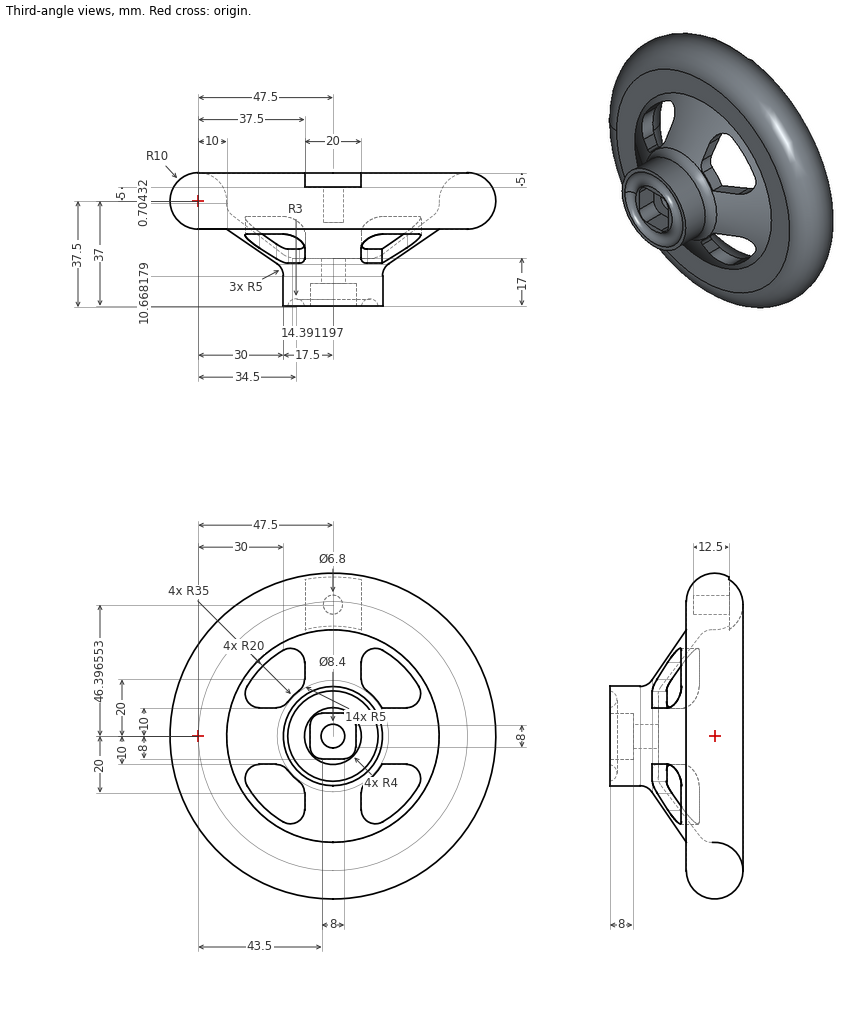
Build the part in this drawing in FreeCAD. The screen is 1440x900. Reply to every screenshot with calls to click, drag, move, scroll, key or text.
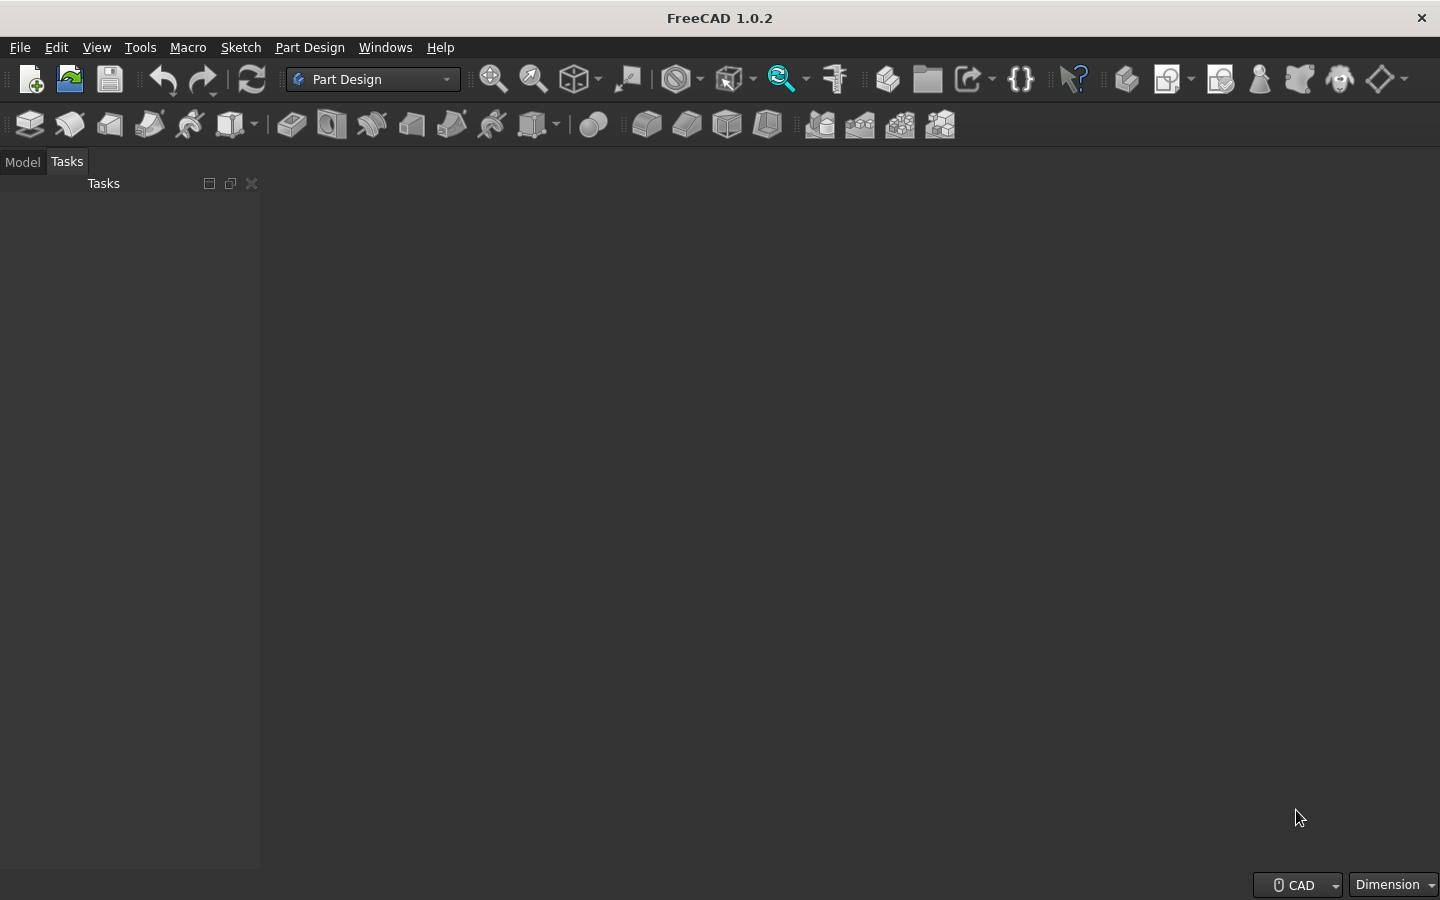
click(30, 80)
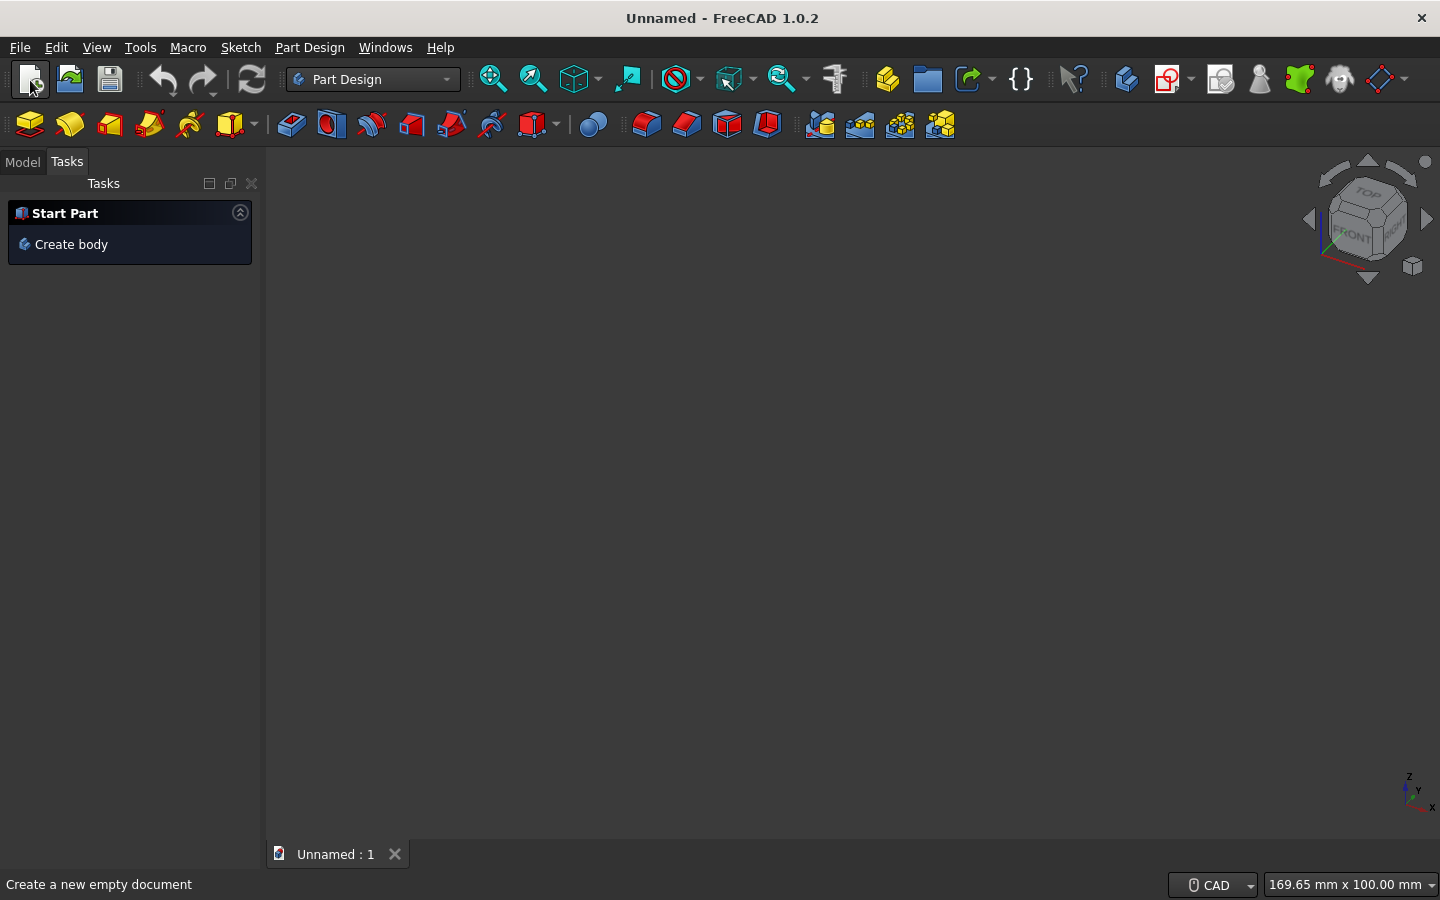
click(1168, 80)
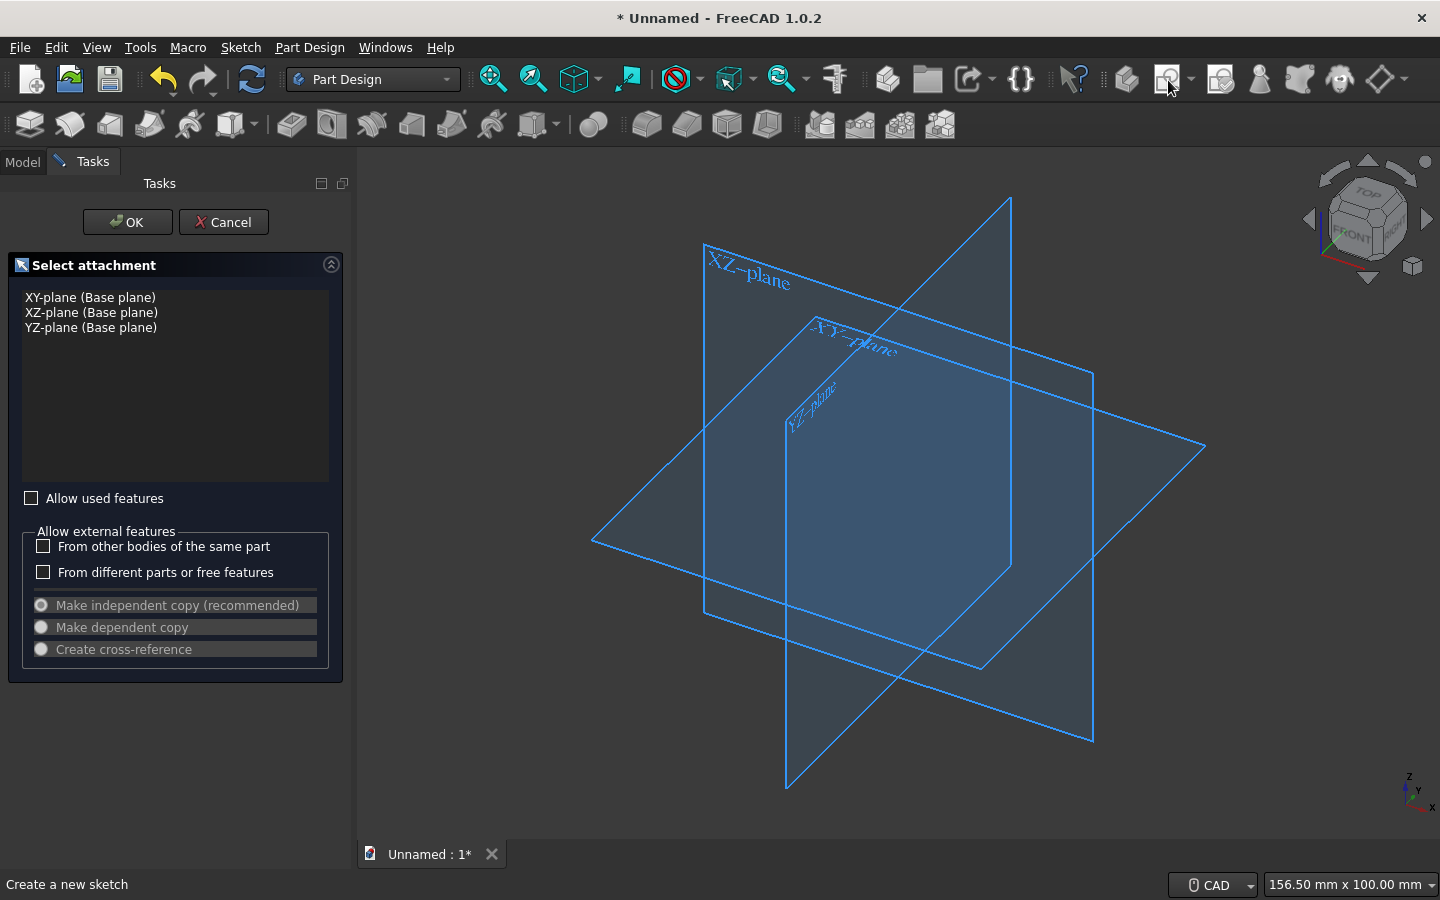
click(82, 298)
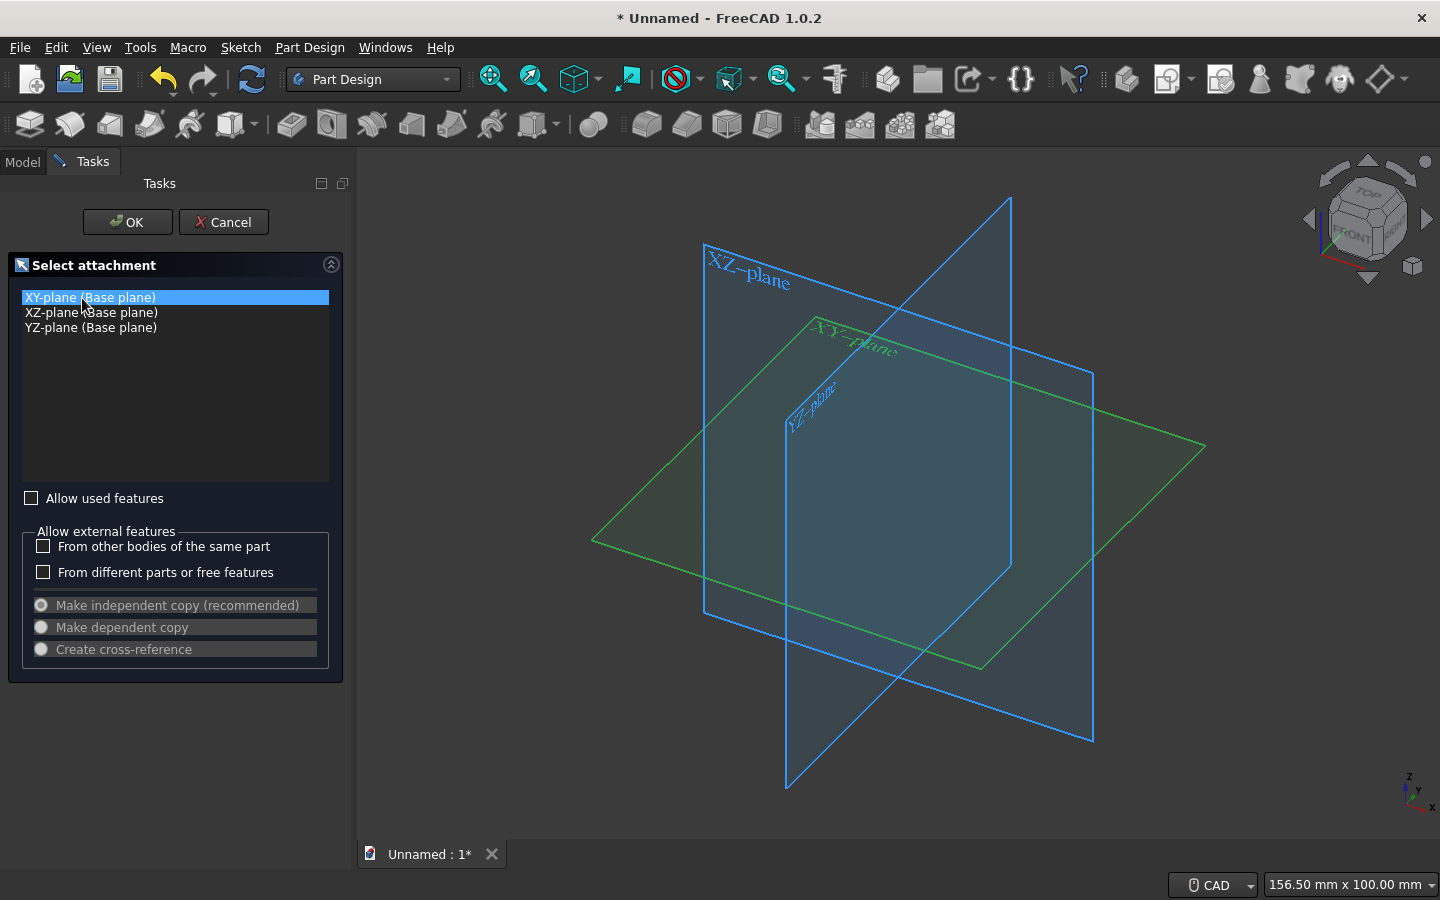
click(128, 222)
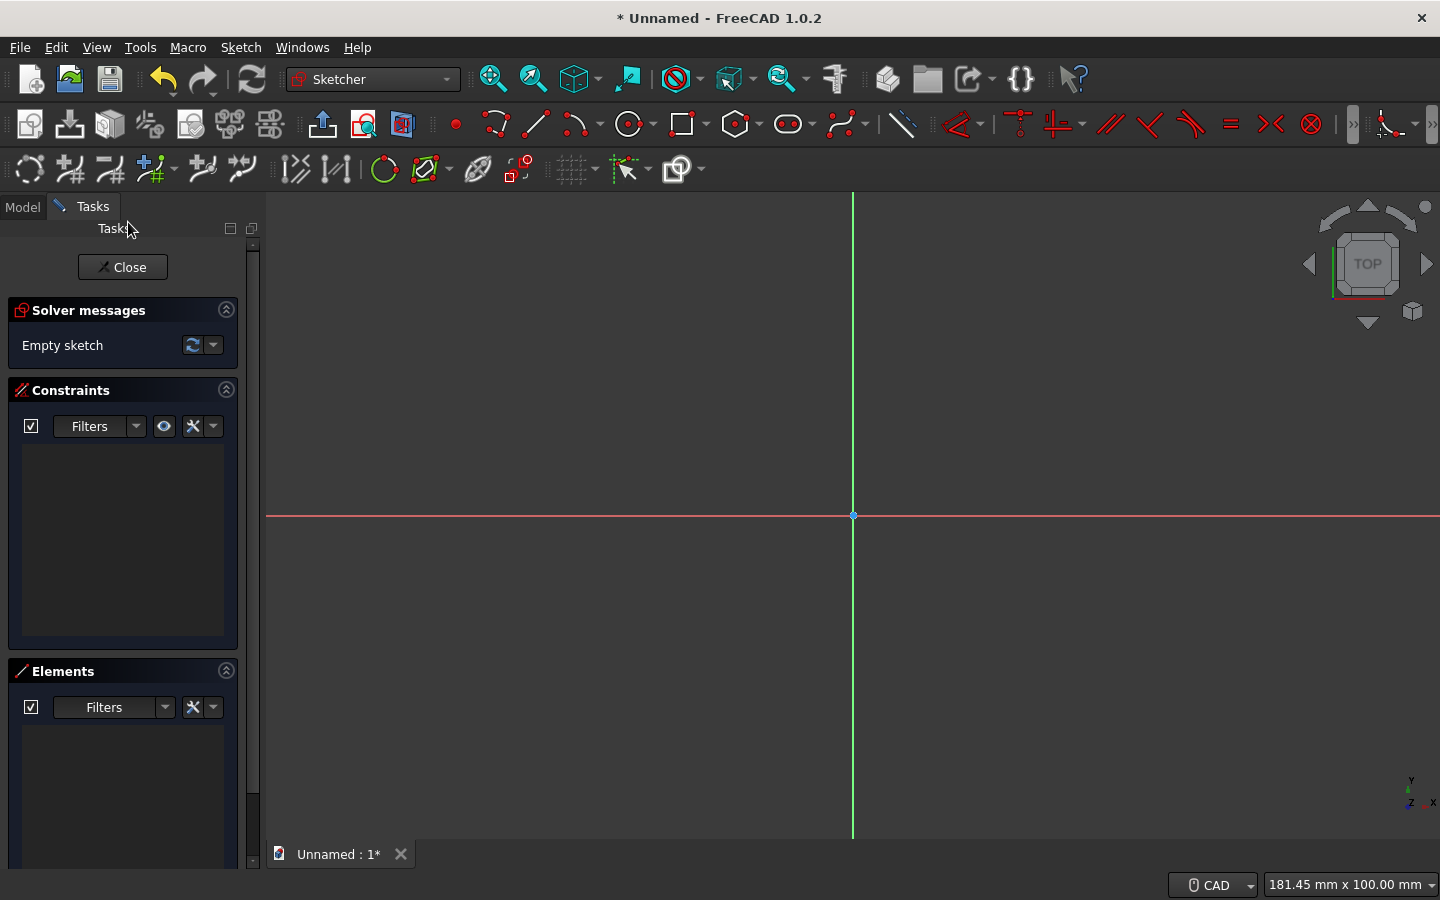
click(496, 124)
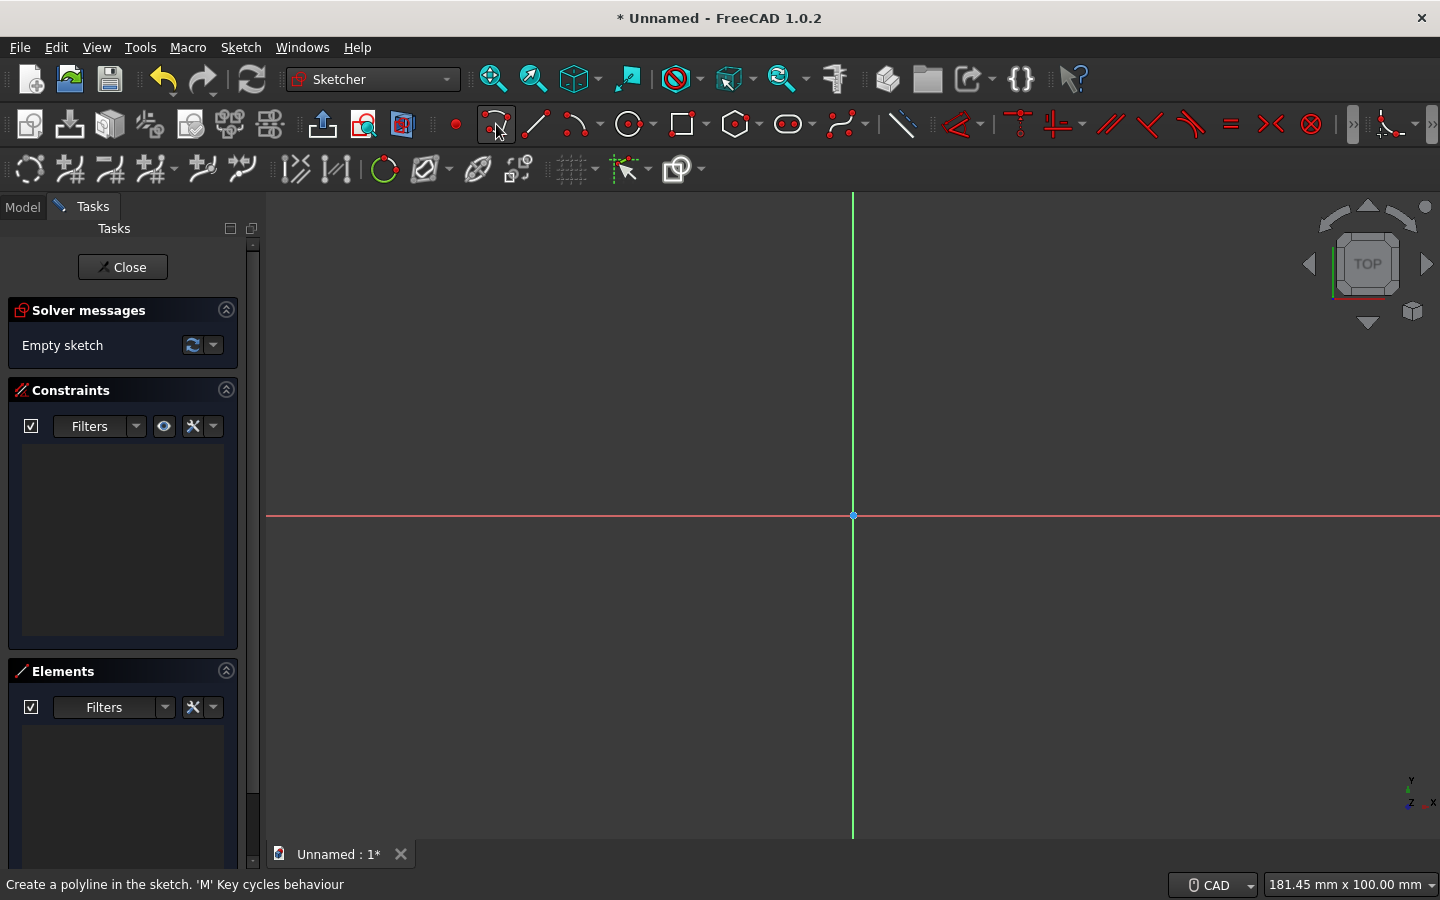
click(853, 580)
click(918, 580)
click(1033, 659)
right_click(1033, 659)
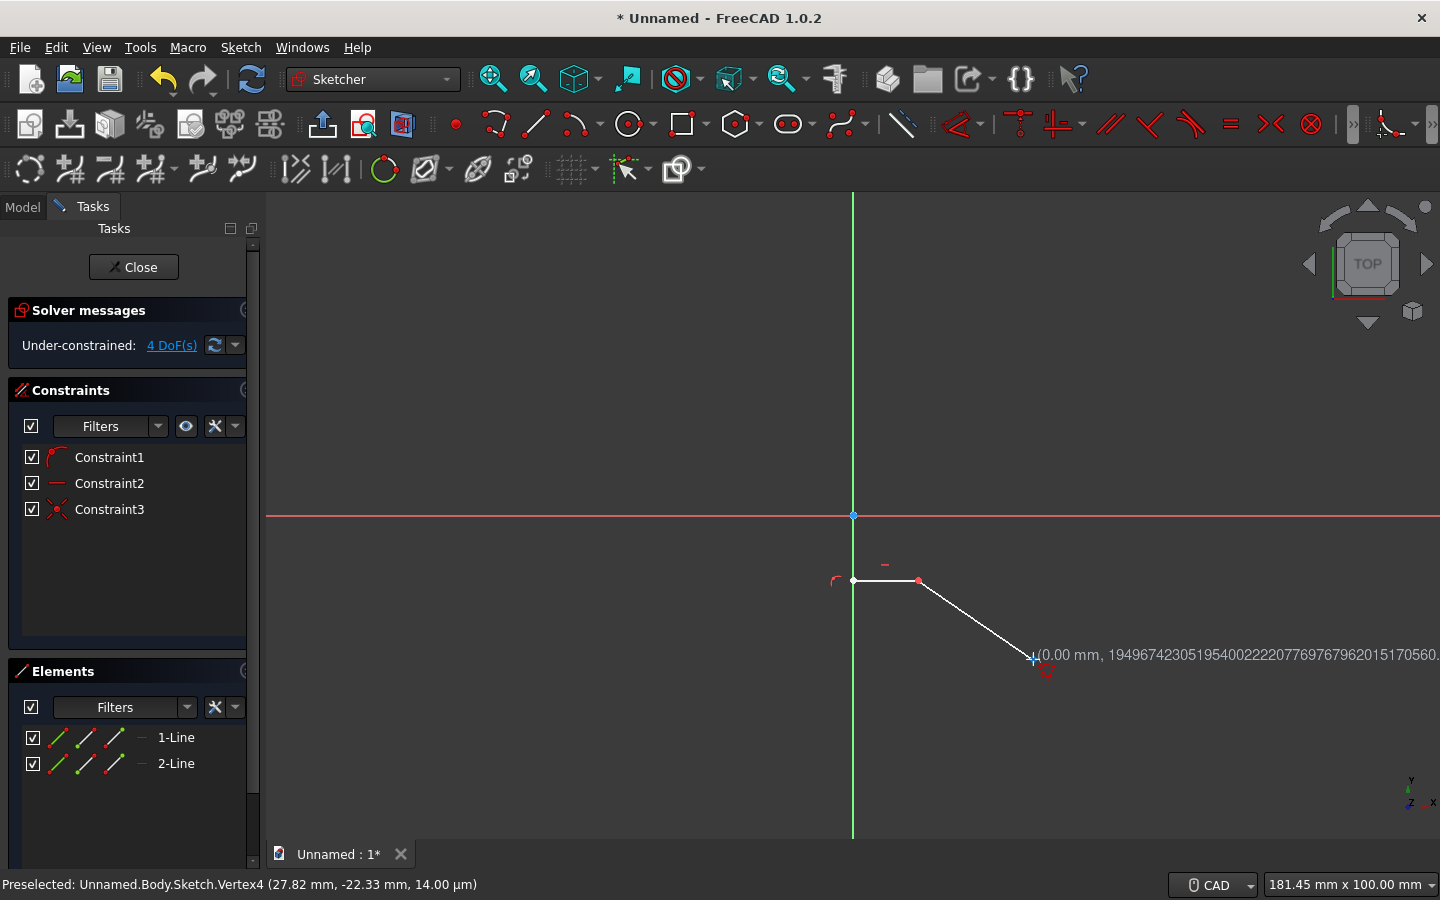
click(1047, 686)
click(1047, 755)
click(1160, 755)
click(1160, 645)
click(1067, 645)
right_click(1067, 645)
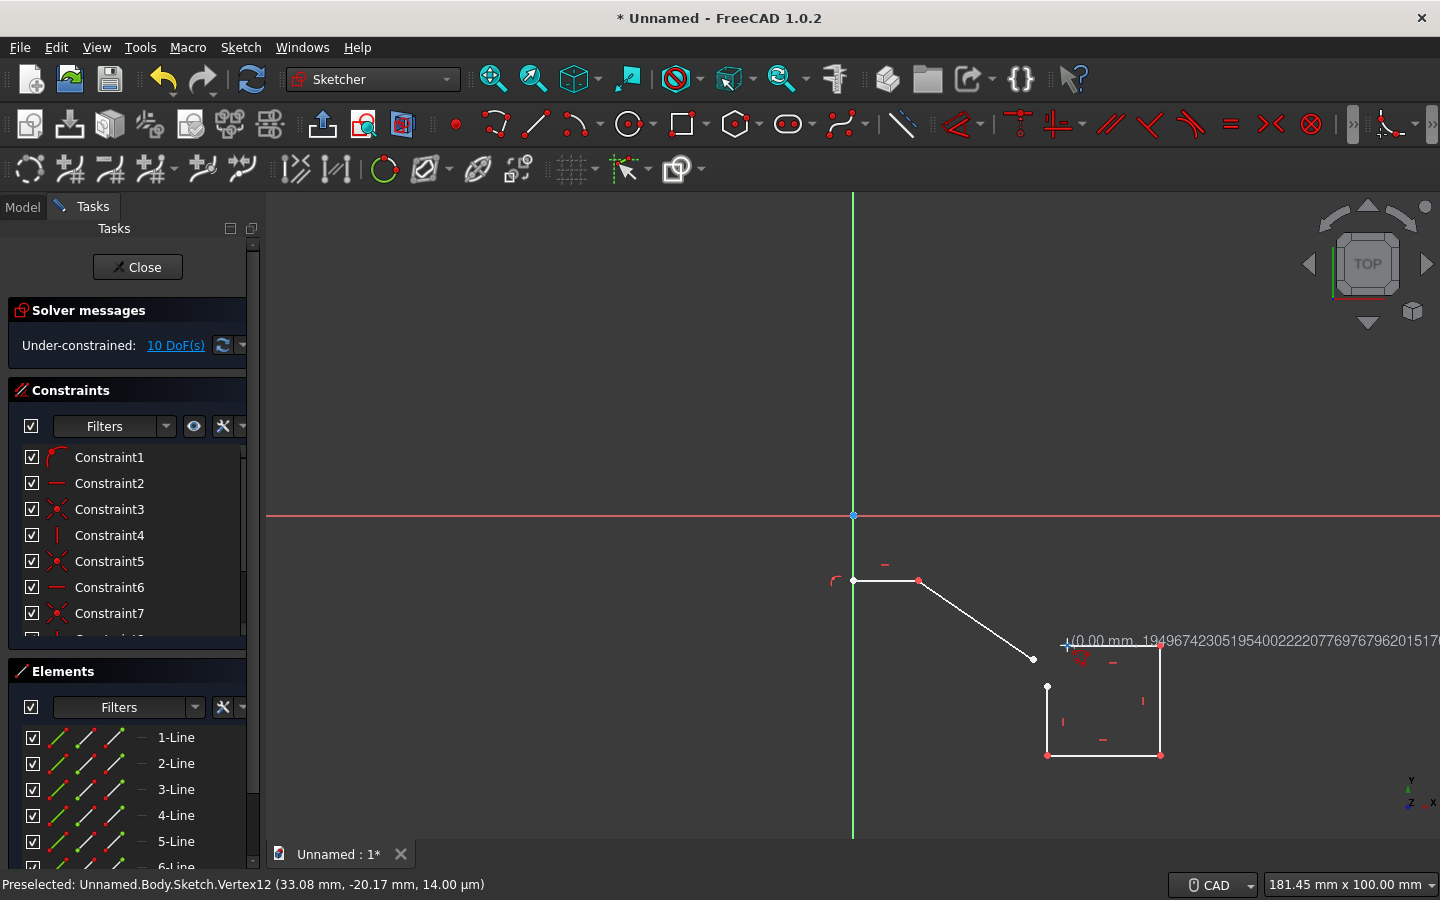
click(536, 124)